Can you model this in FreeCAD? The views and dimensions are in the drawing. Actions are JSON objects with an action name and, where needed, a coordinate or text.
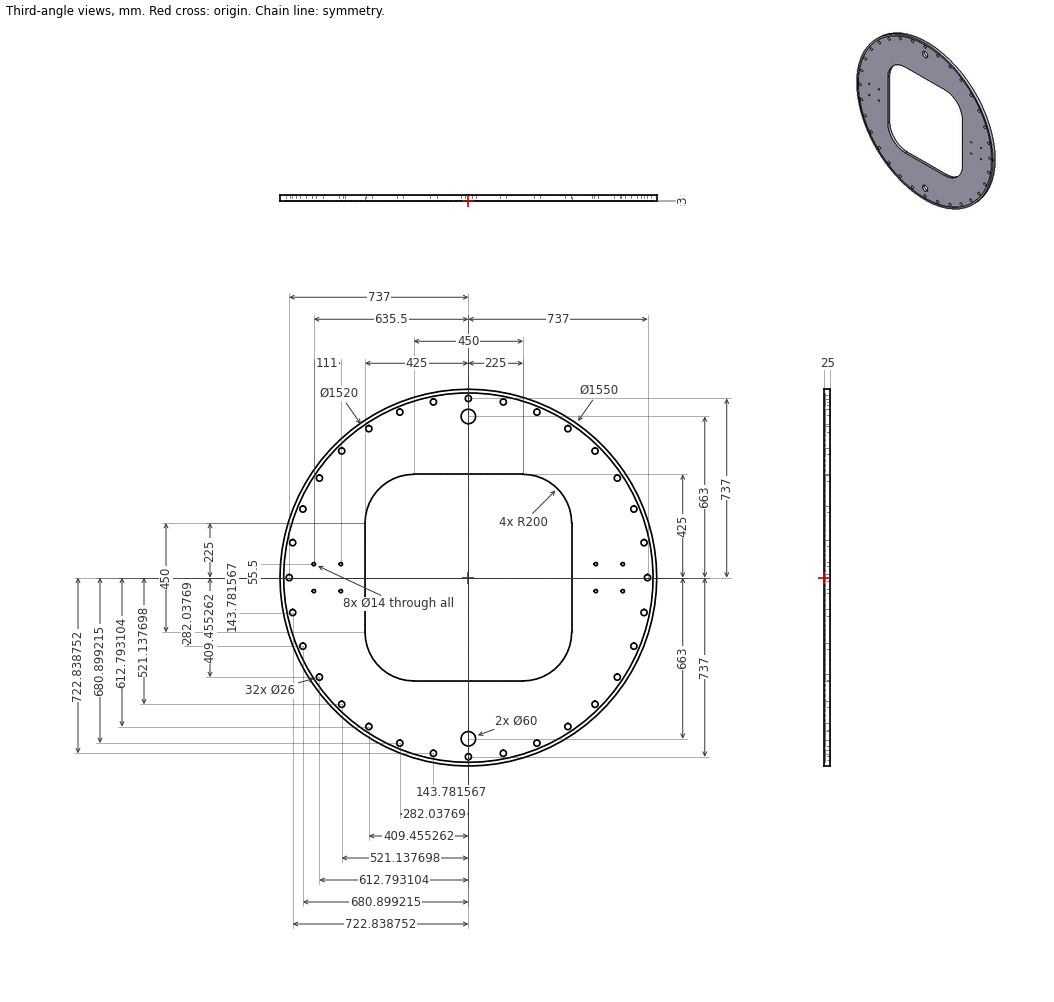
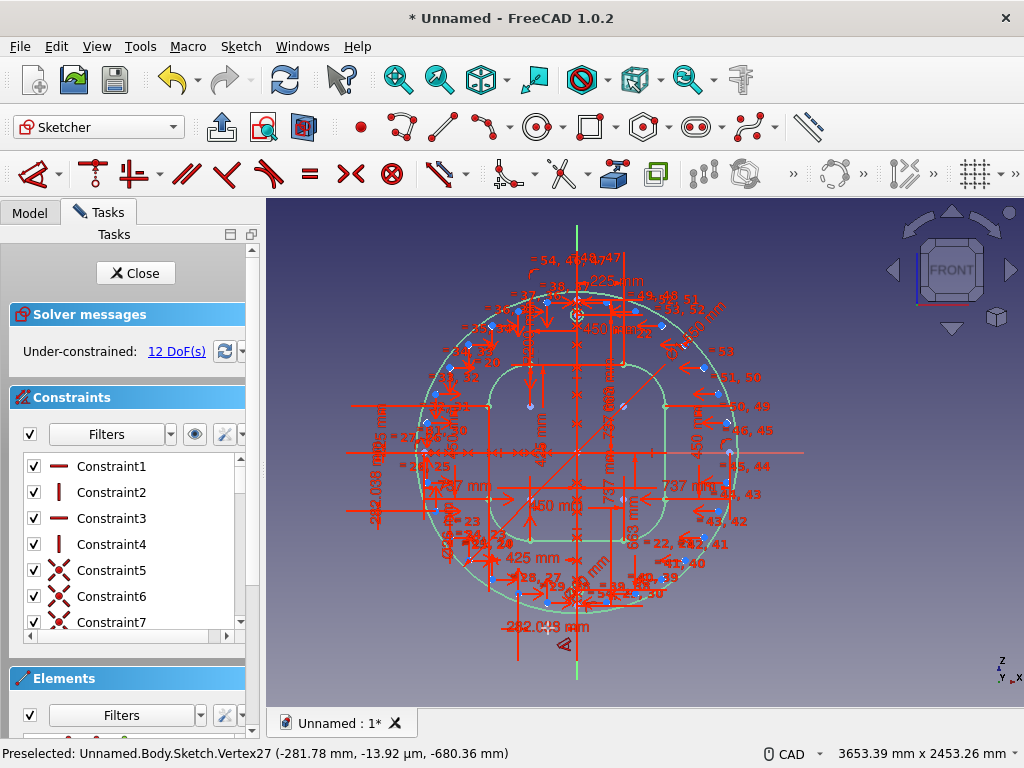
{"action": "left_click", "coordinate": [450, 538]}
{"action": "left_click", "coordinate": [469, 596]}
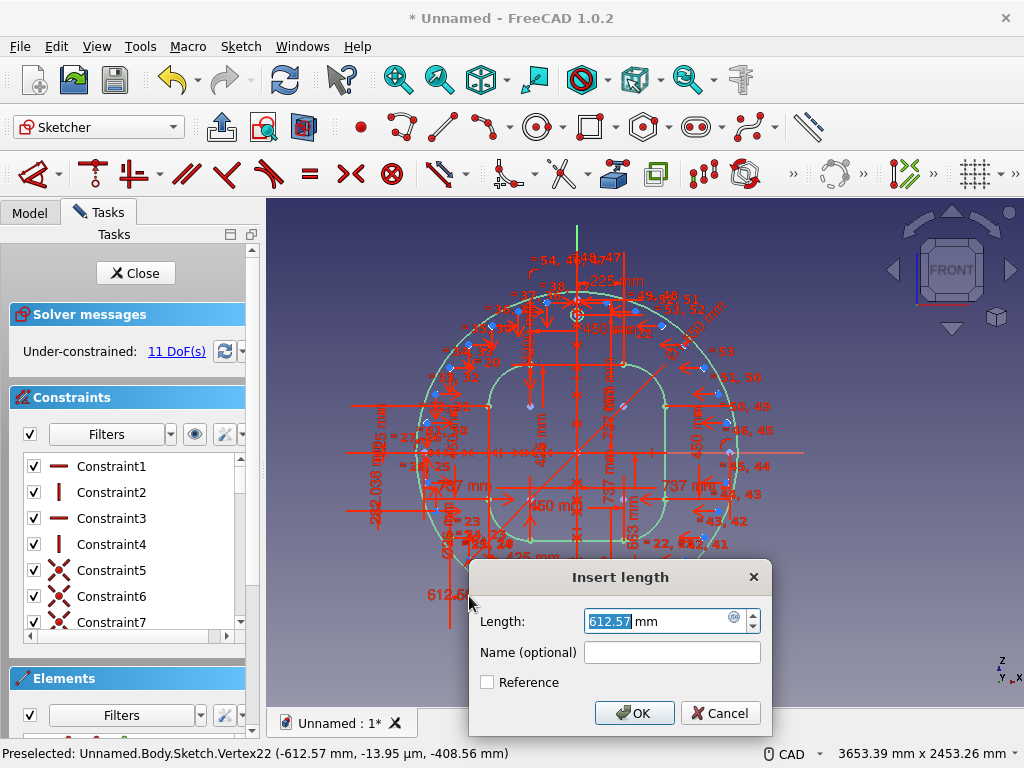
{"action": "type", "text": "612.793104"}
{"action": "key", "text": "Return"}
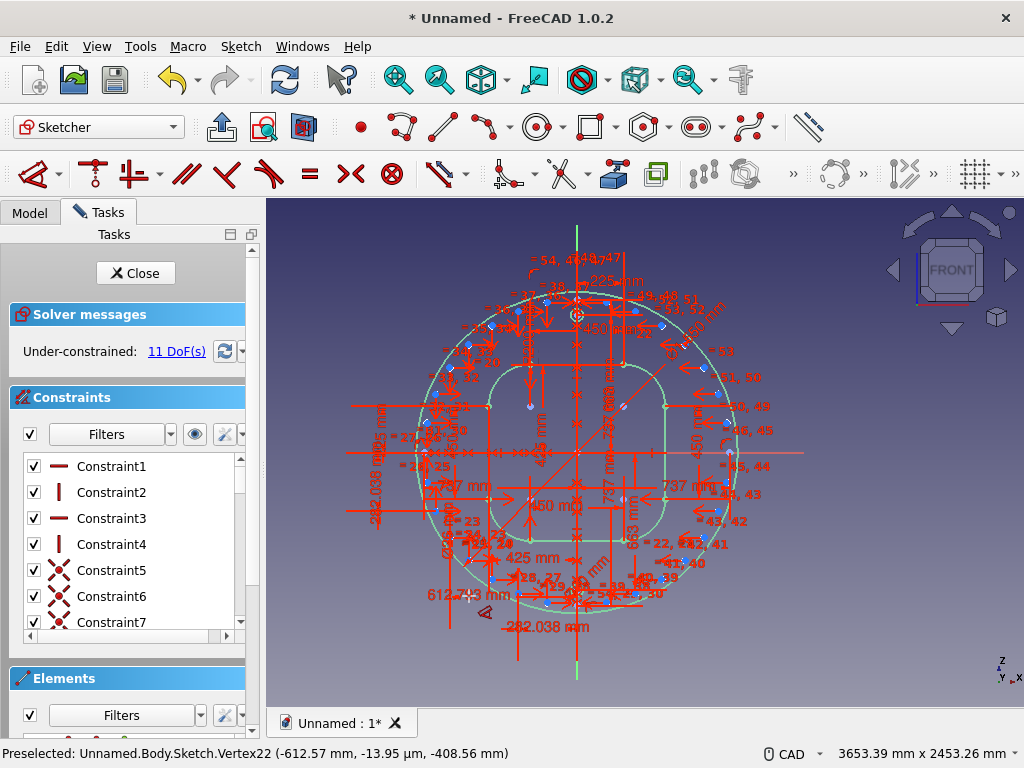
{"action": "left_click", "coordinate": [450, 538]}
{"action": "left_click", "coordinate": [368, 515]}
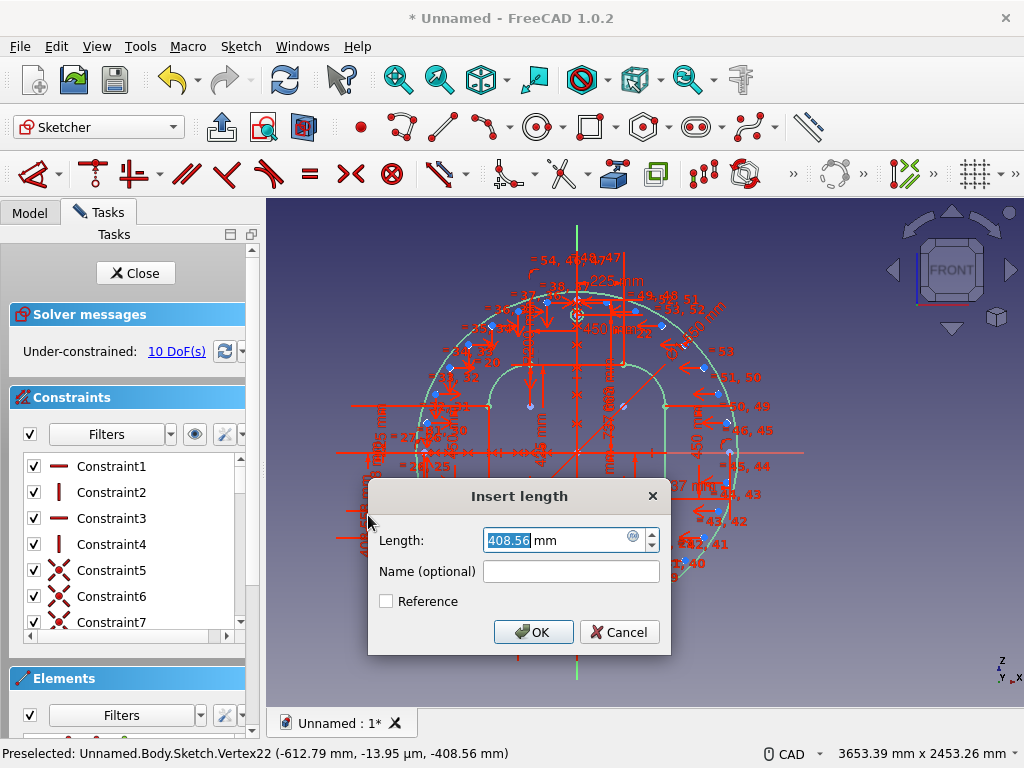
{"action": "type", "text": "409.455262"}
{"action": "key", "text": "Return"}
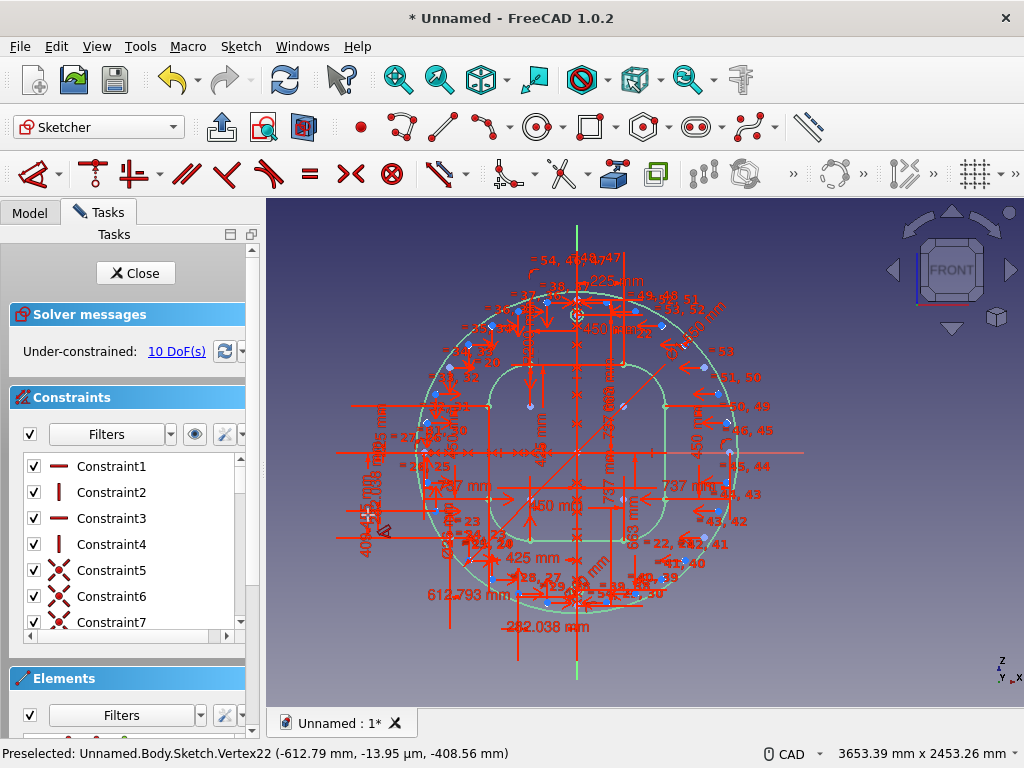
{"action": "left_click", "coordinate": [492, 580]}
{"action": "left_click", "coordinate": [535, 419]}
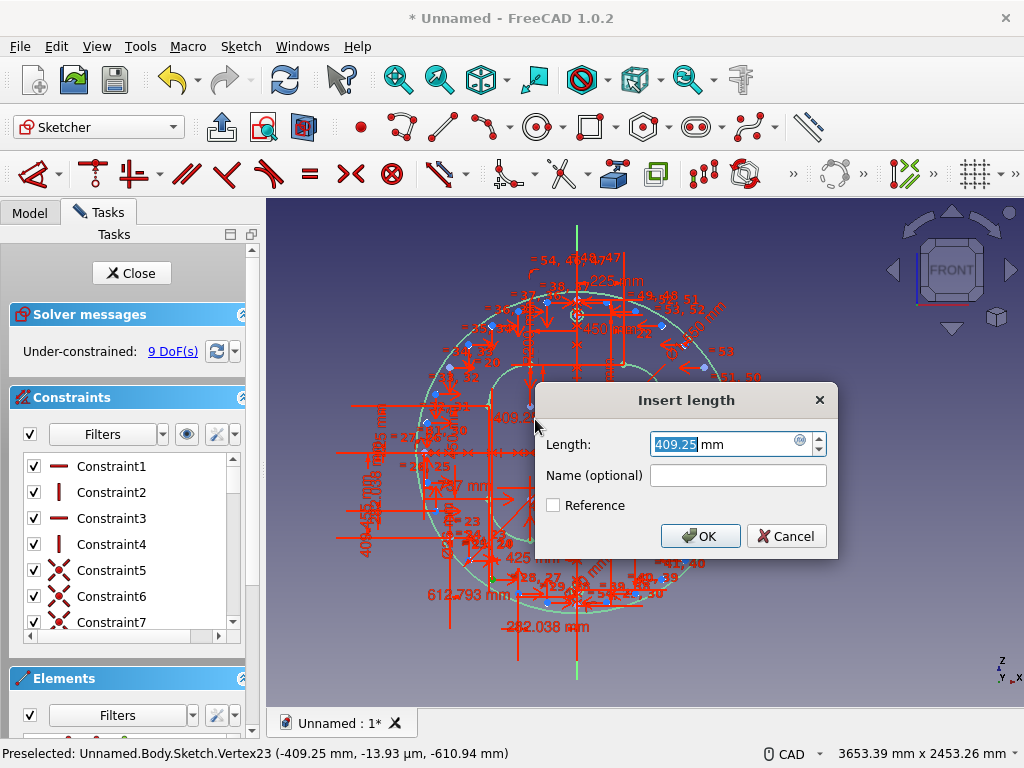
{"action": "type", "text": "409.455262"}
{"action": "key", "text": "Return"}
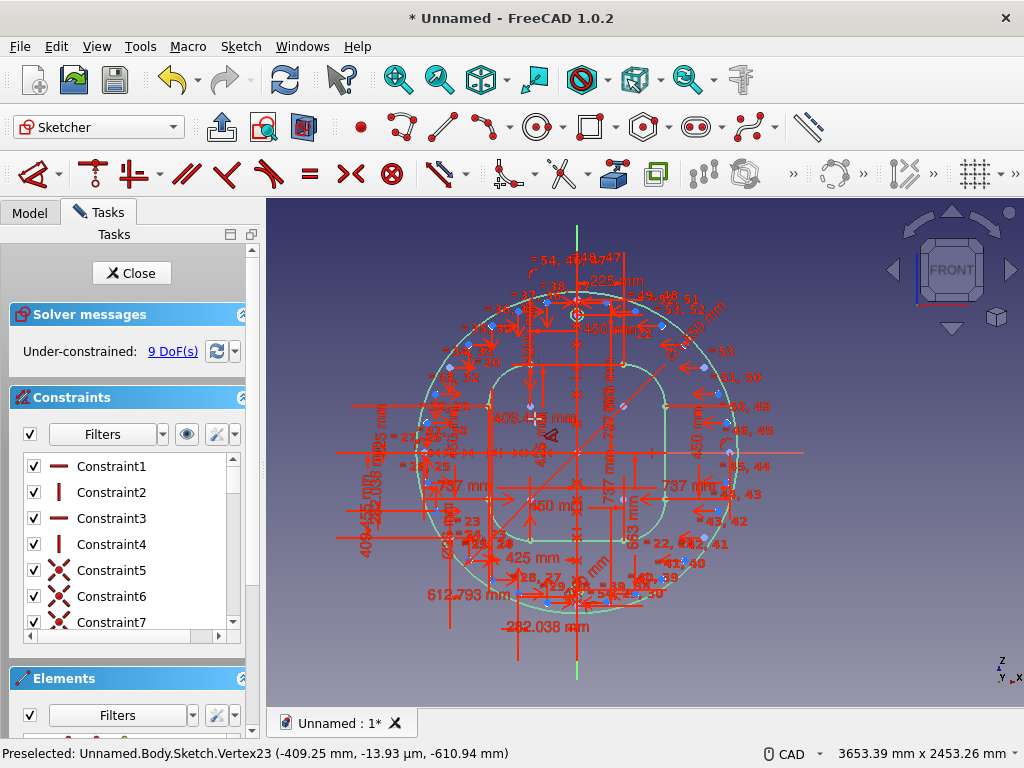
{"action": "left_click", "coordinate": [492, 580]}
{"action": "left_click", "coordinate": [434, 560]}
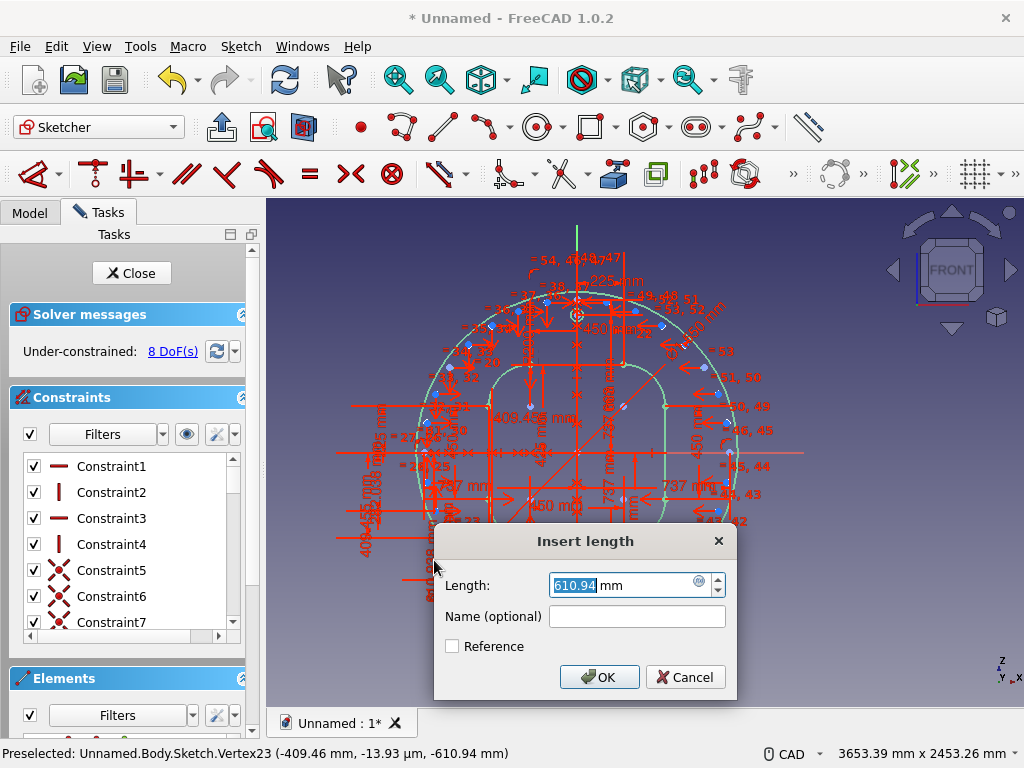
{"action": "type", "text": "612.793104"}
{"action": "key", "text": "Return"}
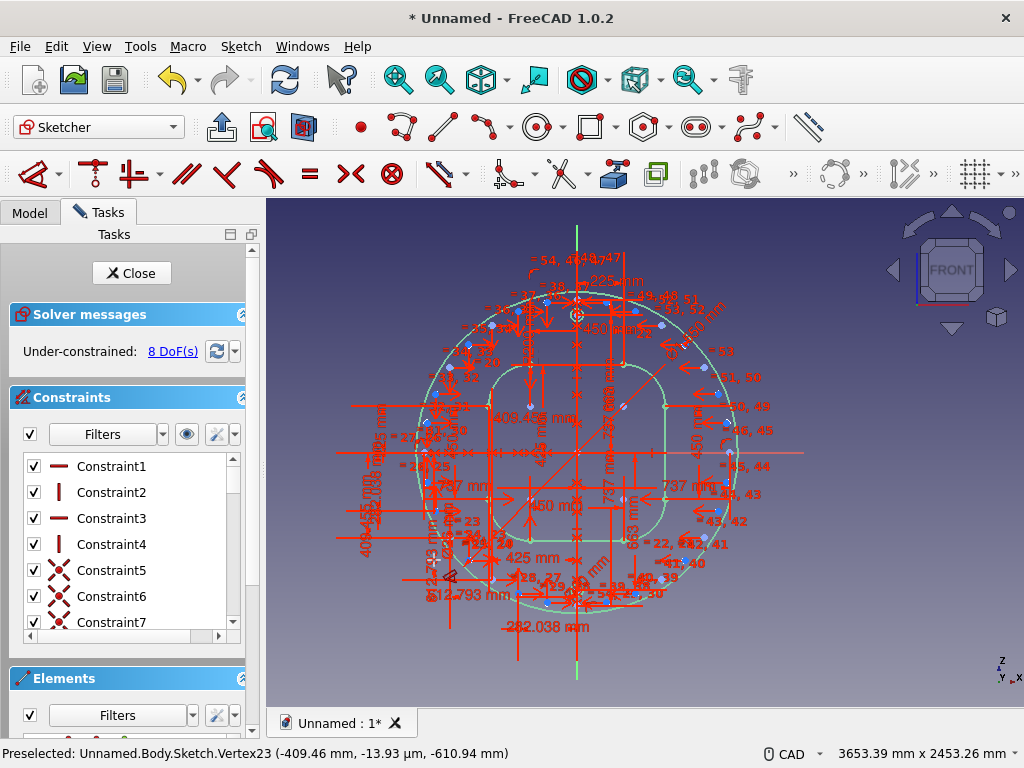
{"action": "left_click", "coordinate": [469, 561]}
{"action": "left_click", "coordinate": [523, 395]}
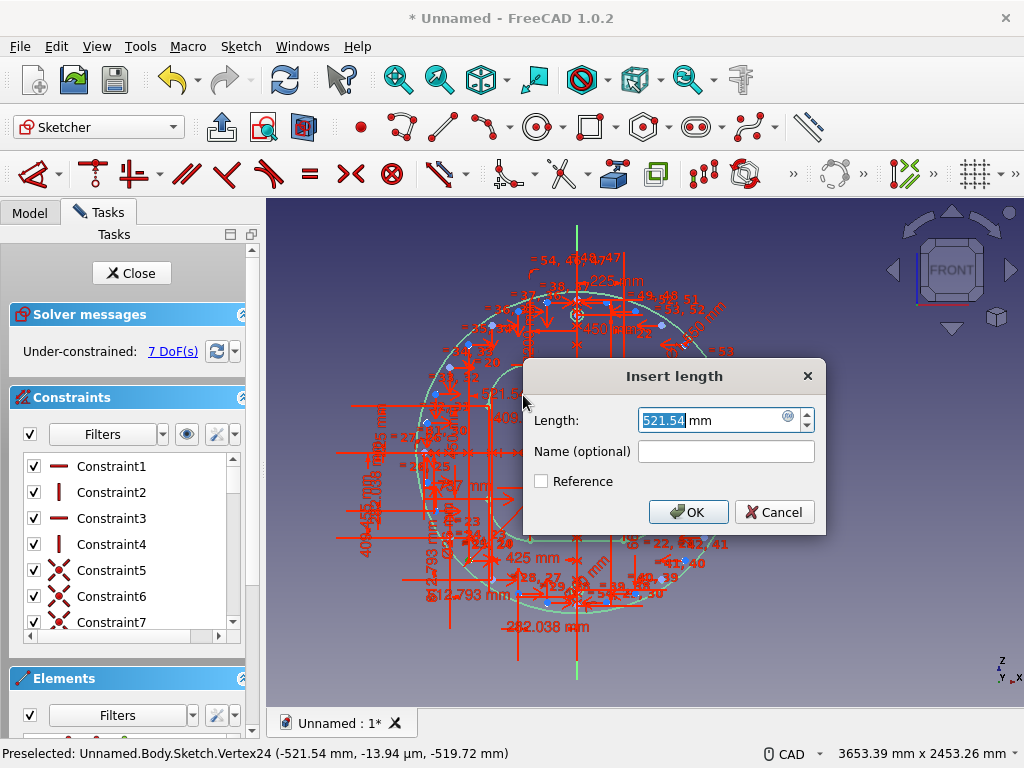
{"action": "type", "text": "521.137698"}
{"action": "key", "text": "Return"}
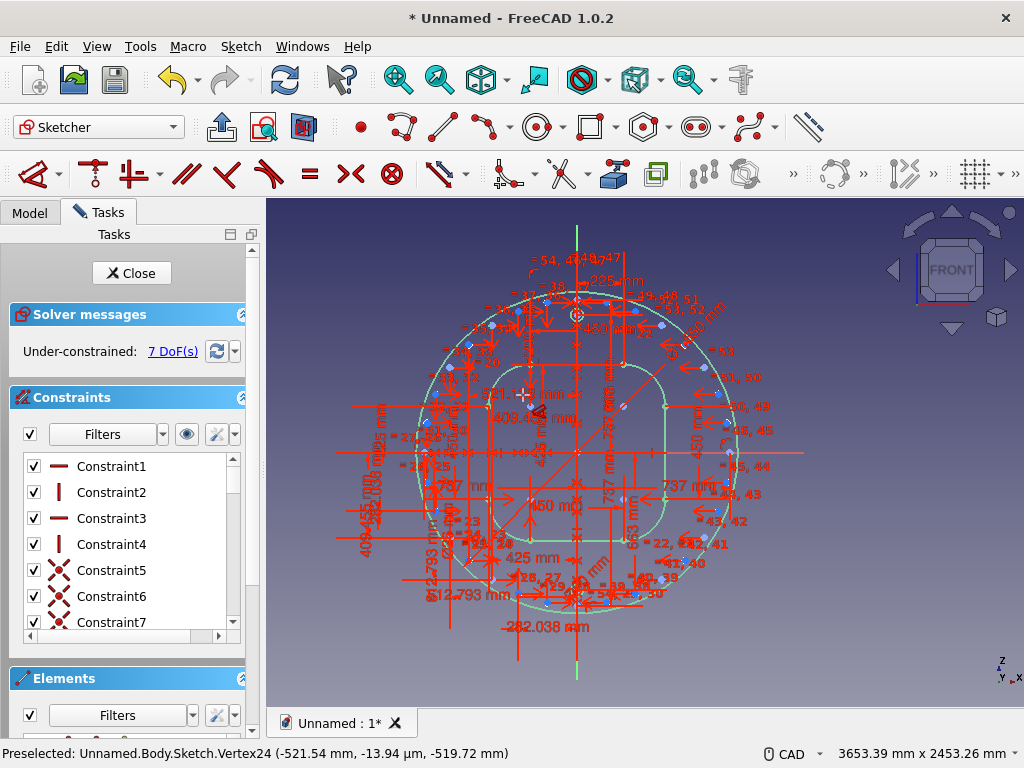
{"action": "left_click", "coordinate": [469, 561]}
{"action": "left_click", "coordinate": [659, 544]}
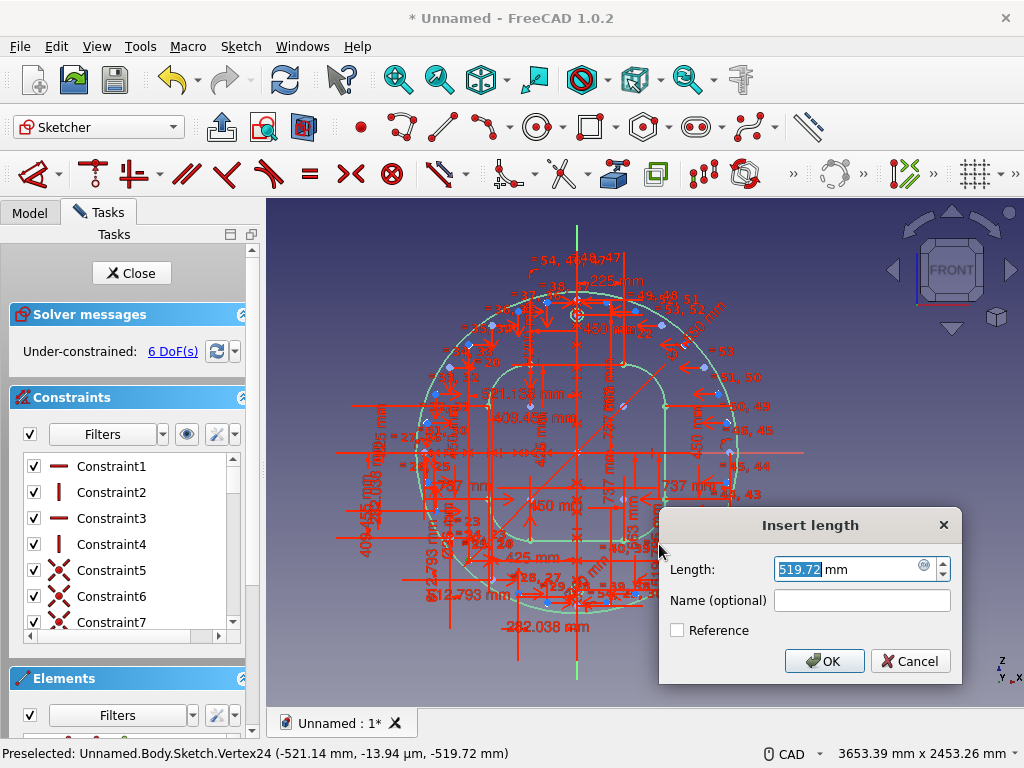
{"action": "type", "text": "521.137698"}
{"action": "key", "text": "Return"}